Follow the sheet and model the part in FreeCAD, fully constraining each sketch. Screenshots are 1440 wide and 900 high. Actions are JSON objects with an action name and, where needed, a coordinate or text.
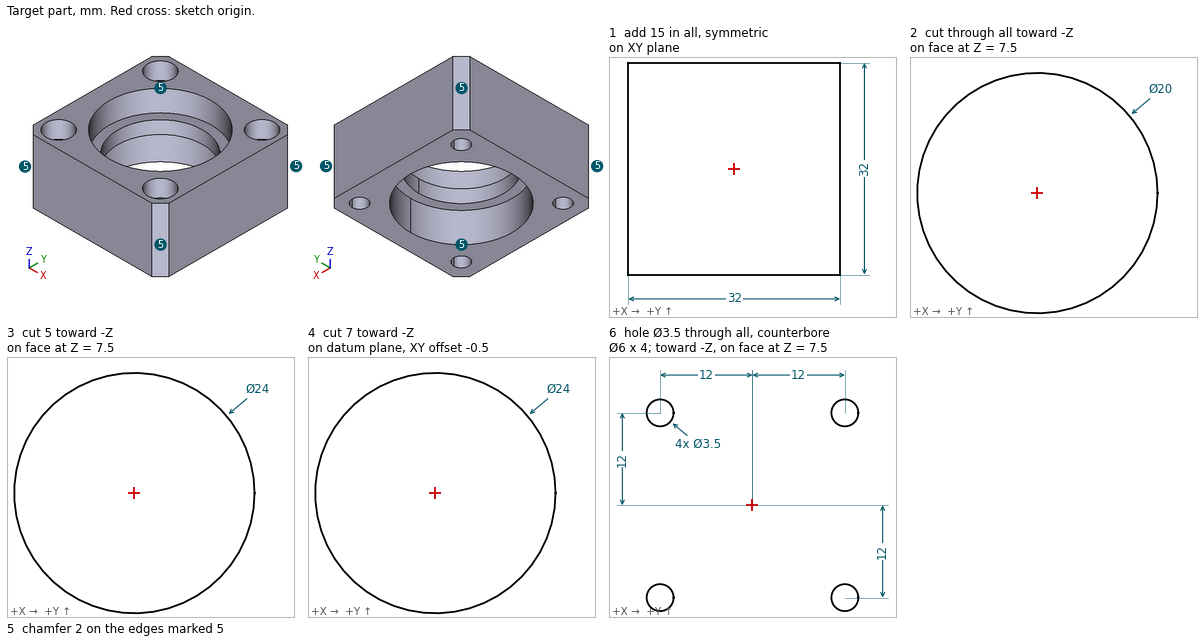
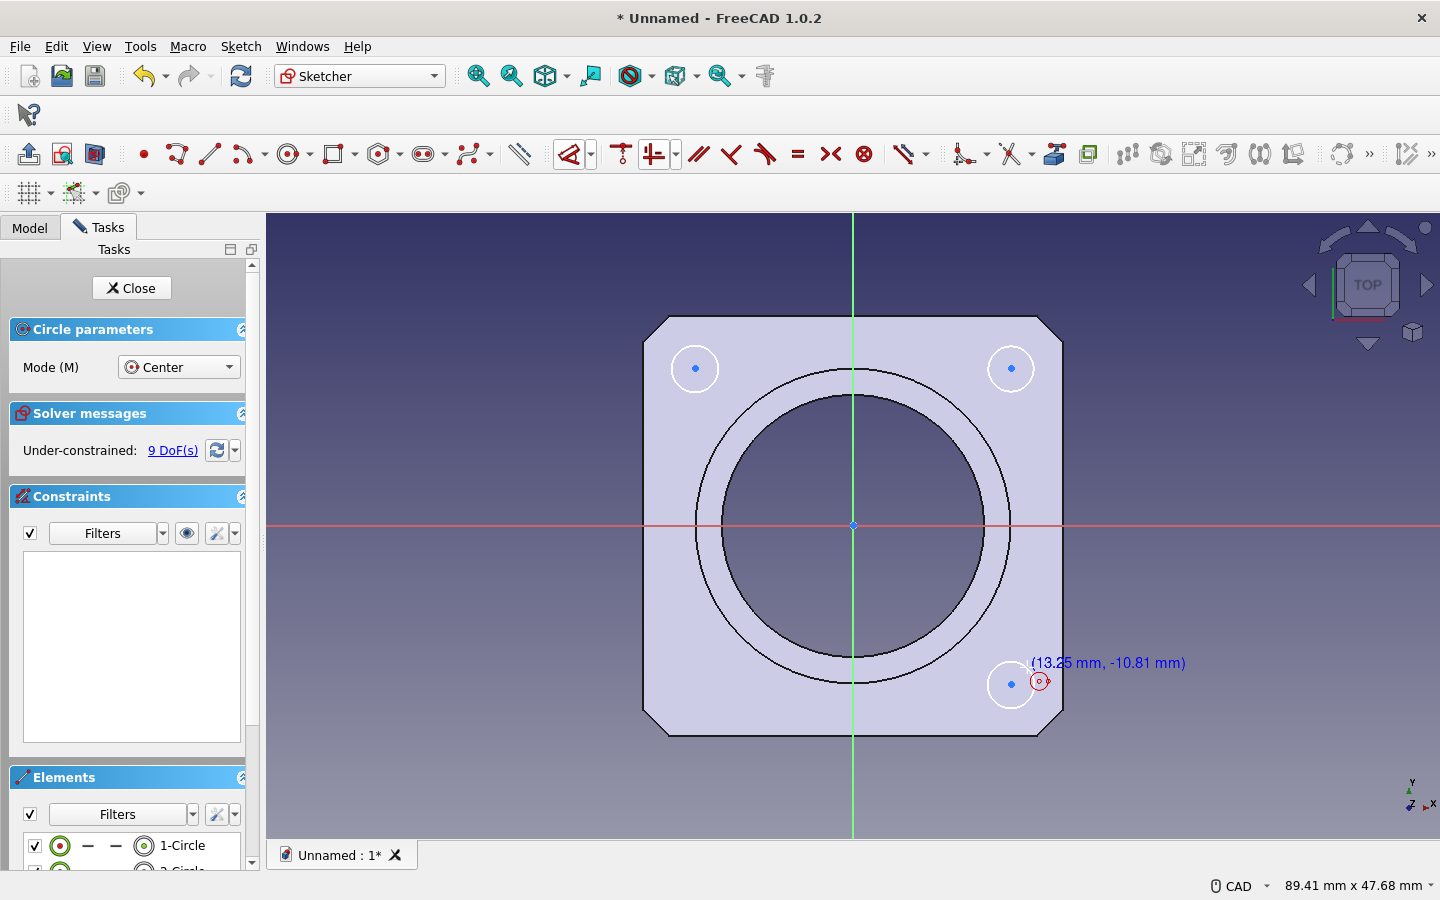
{"action": "left_click", "coordinate": [695, 684]}
{"action": "left_click", "coordinate": [712, 667]}
{"action": "key", "text": "Escape"}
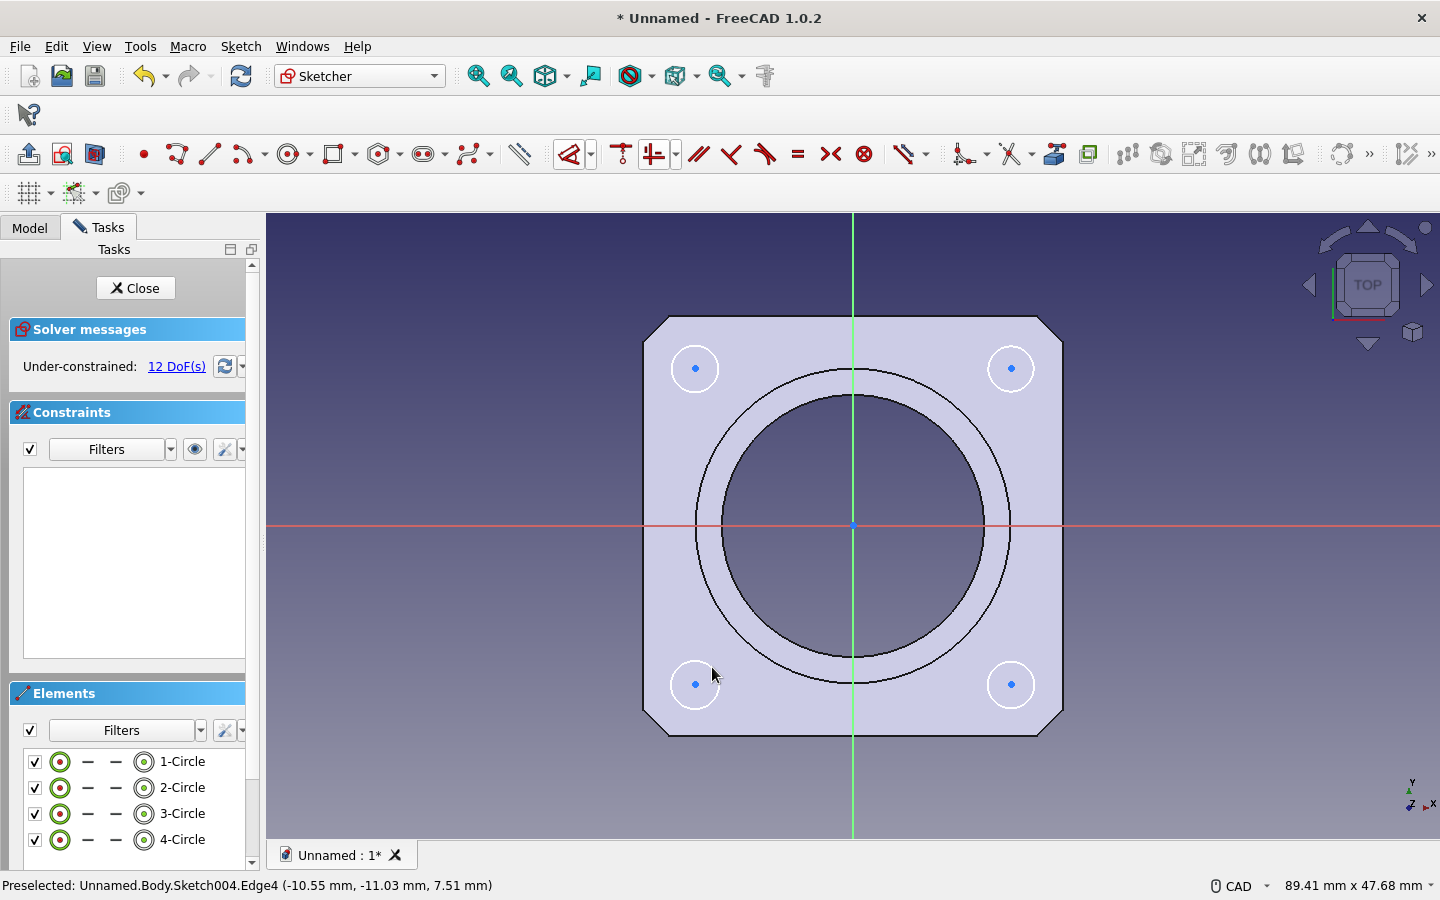
{"action": "left_click", "coordinate": [711, 352]}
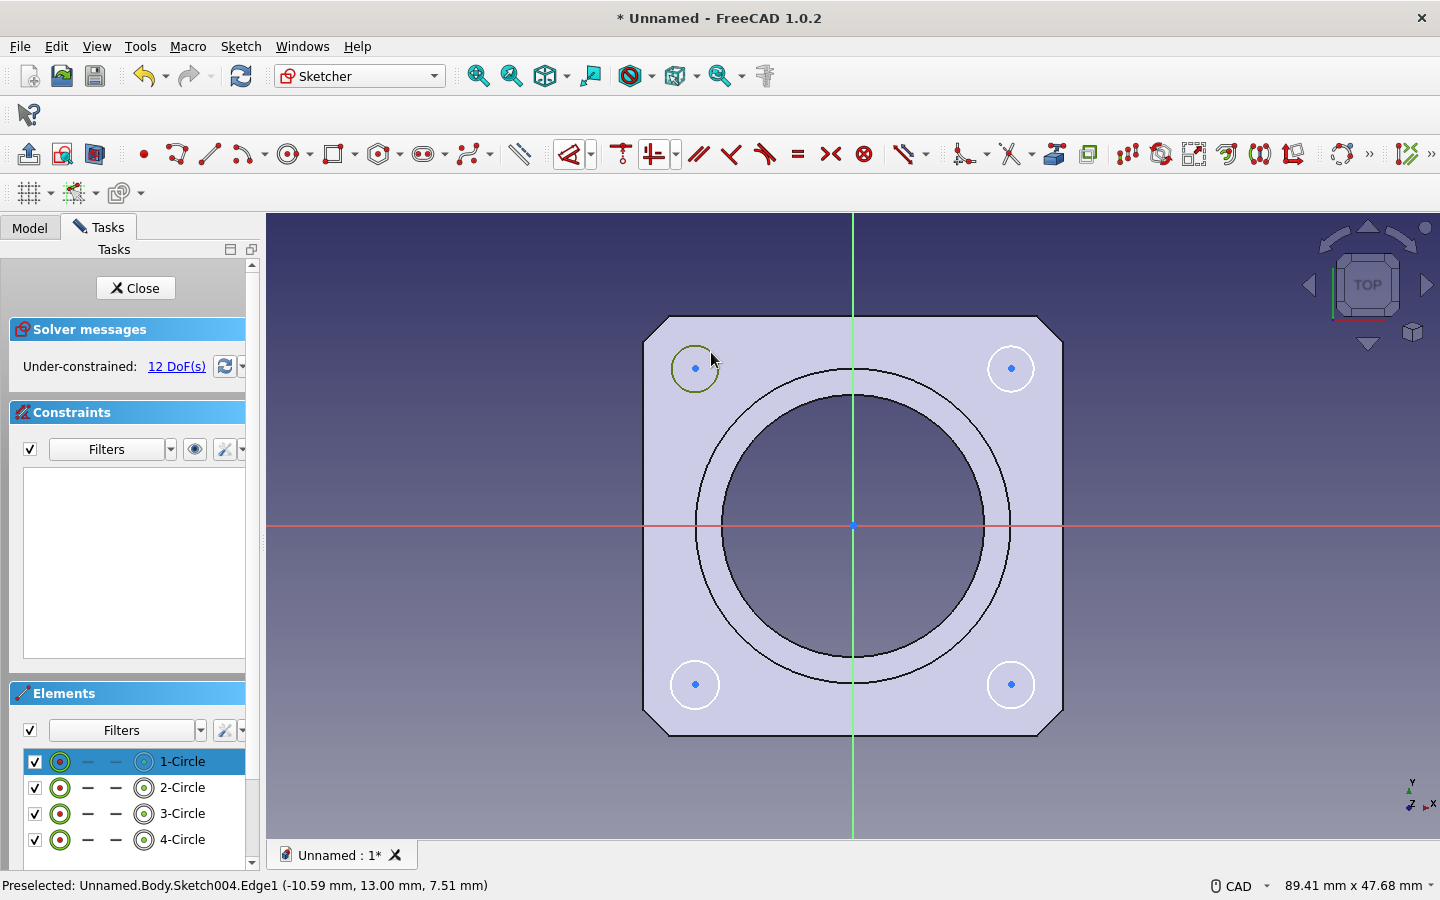
{"action": "left_click", "coordinate": [1027, 353]}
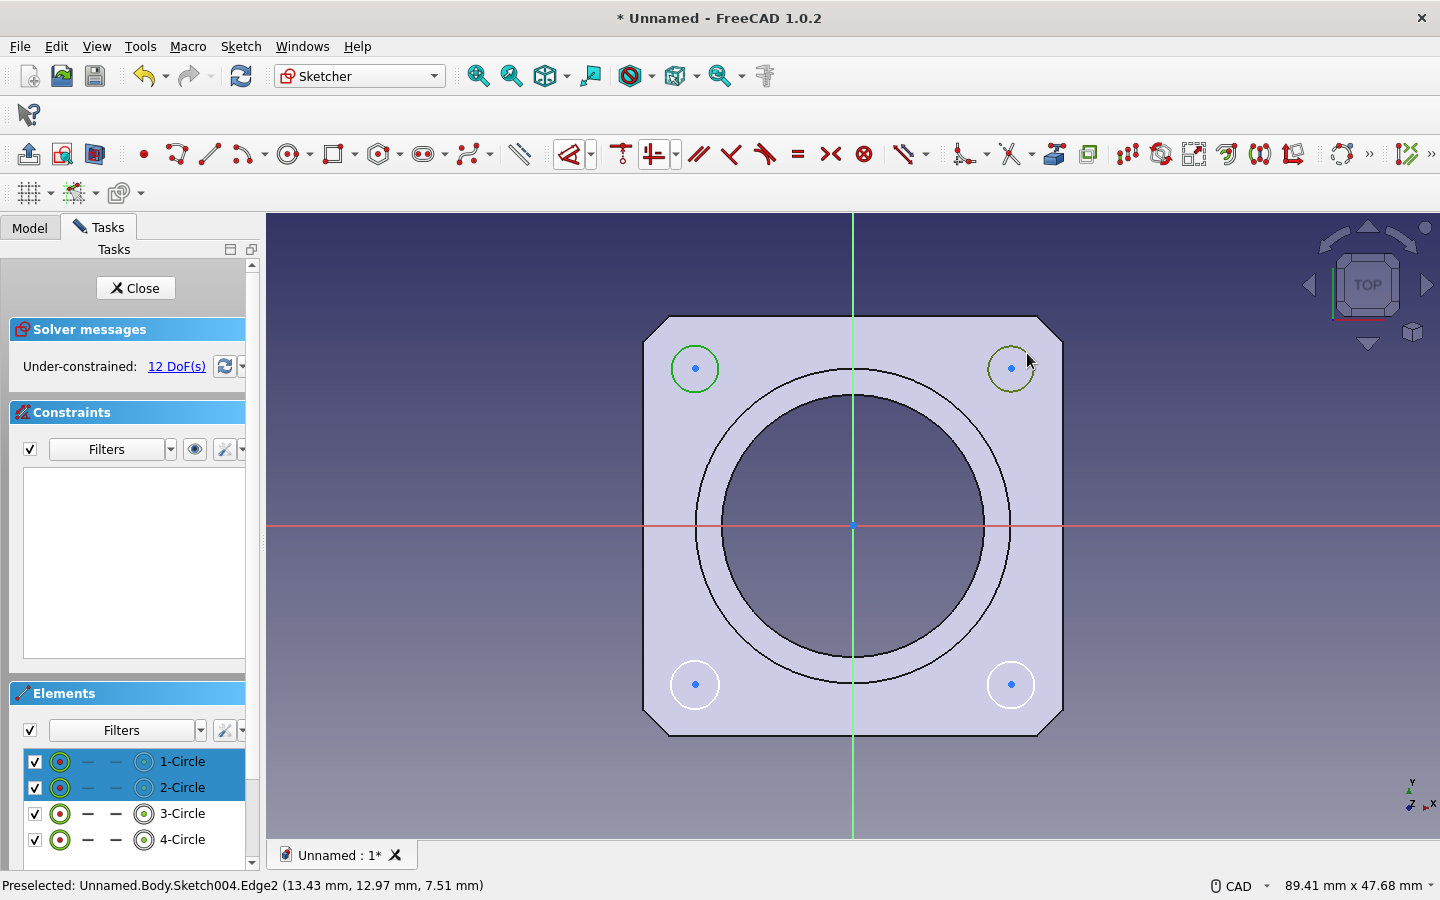
{"action": "left_click", "coordinate": [1027, 668]}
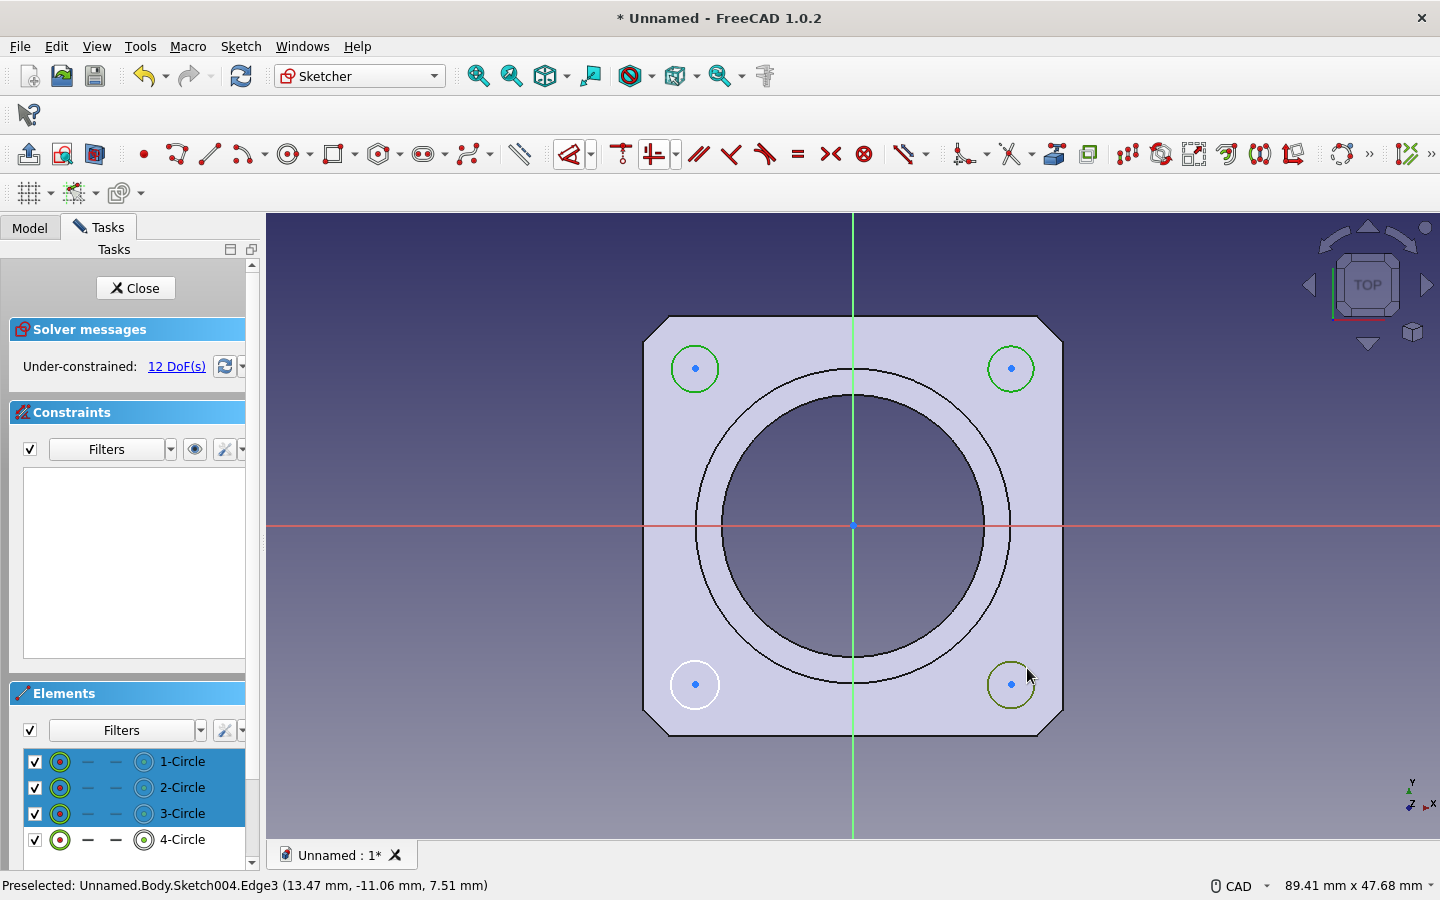
{"action": "left_click", "coordinate": [712, 668]}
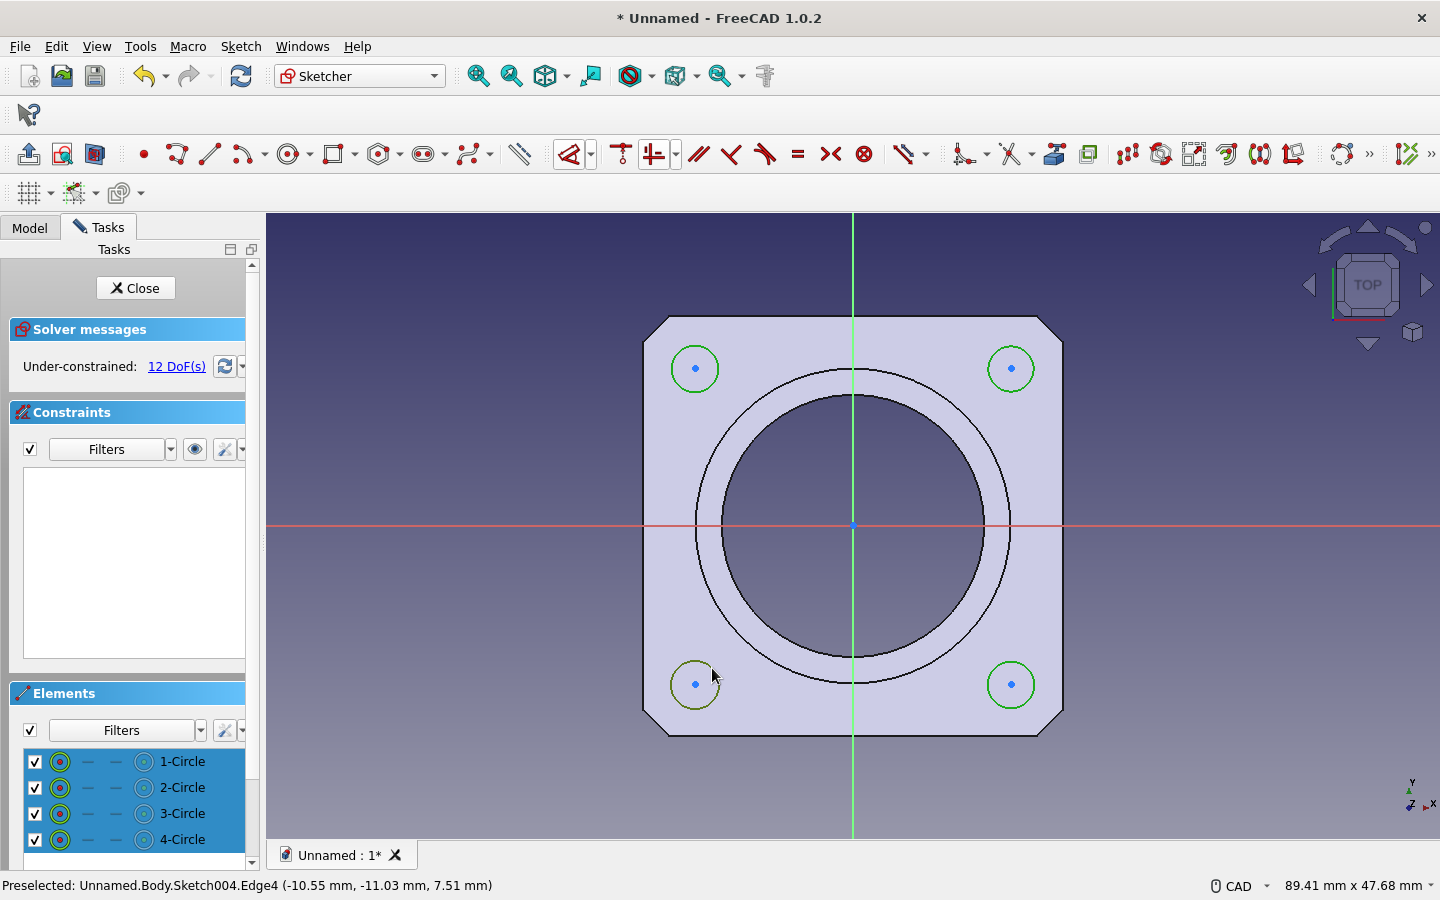
{"action": "left_click", "coordinate": [798, 154]}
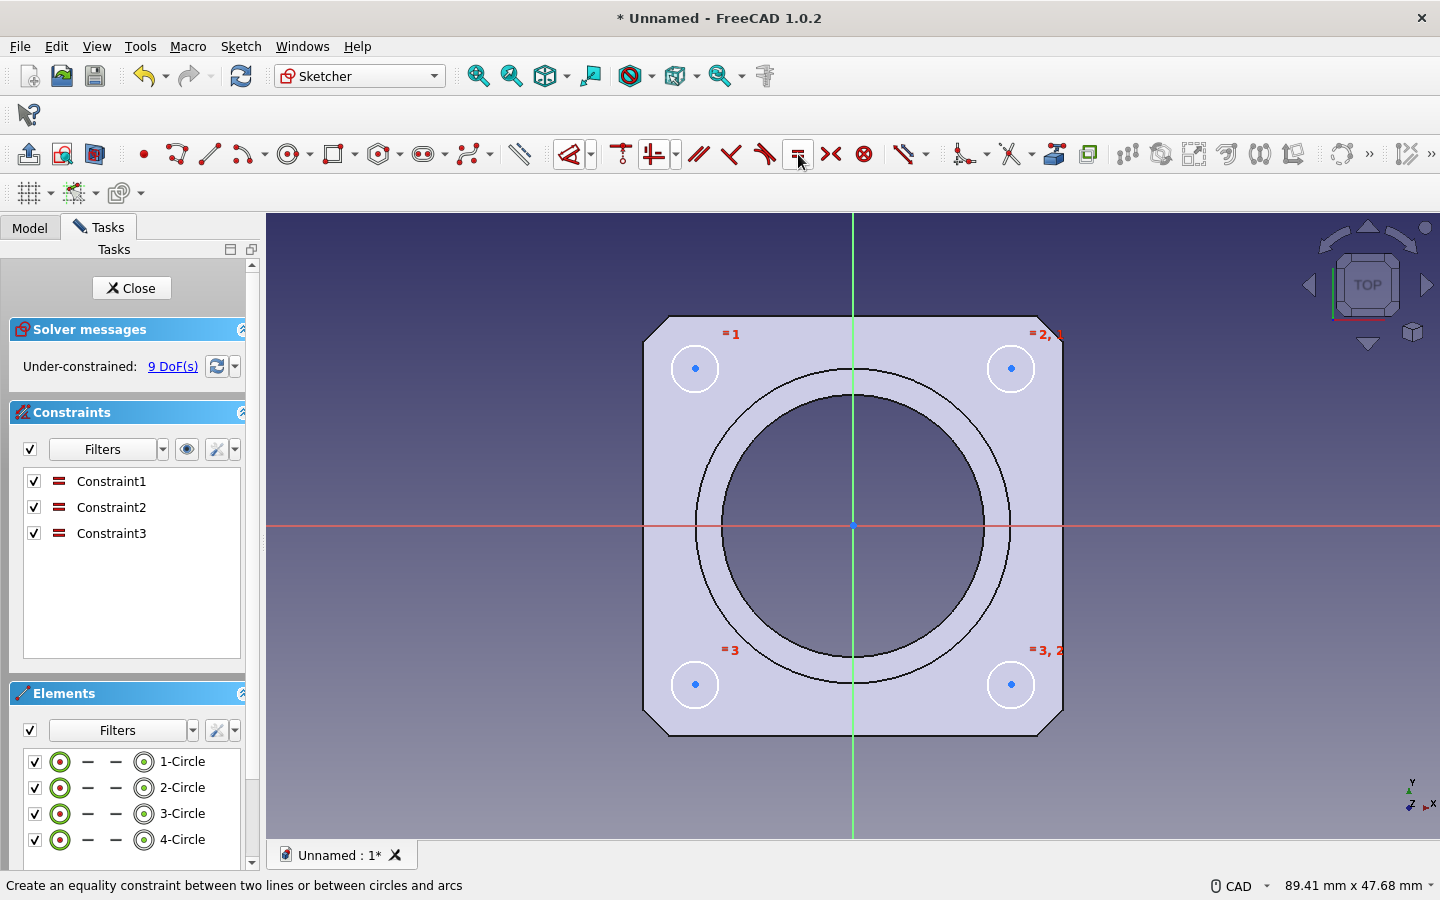
{"action": "left_click", "coordinate": [695, 369]}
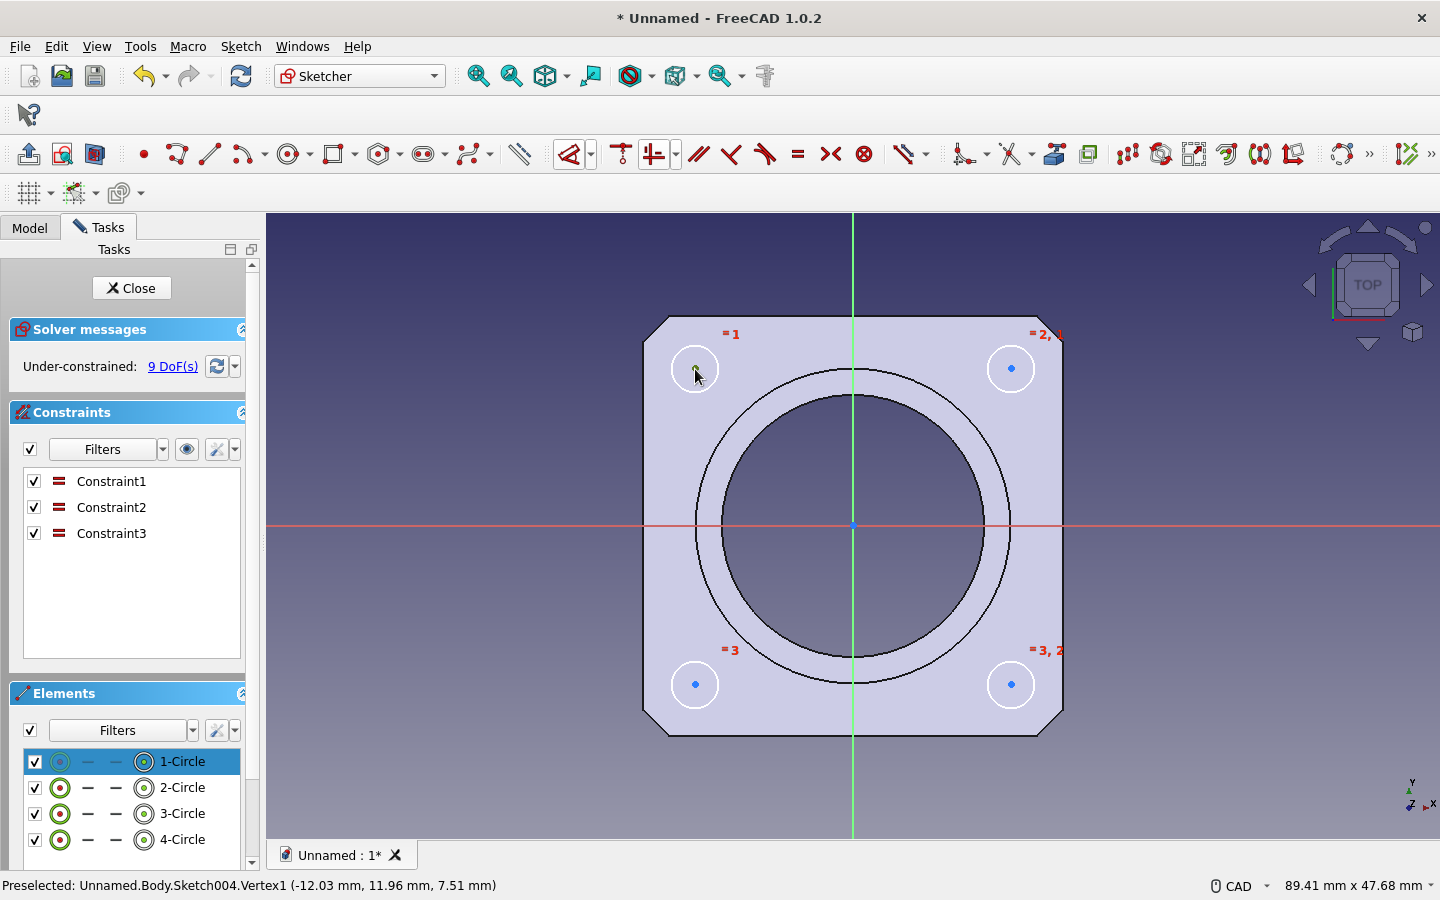
{"action": "left_click", "coordinate": [1011, 369]}